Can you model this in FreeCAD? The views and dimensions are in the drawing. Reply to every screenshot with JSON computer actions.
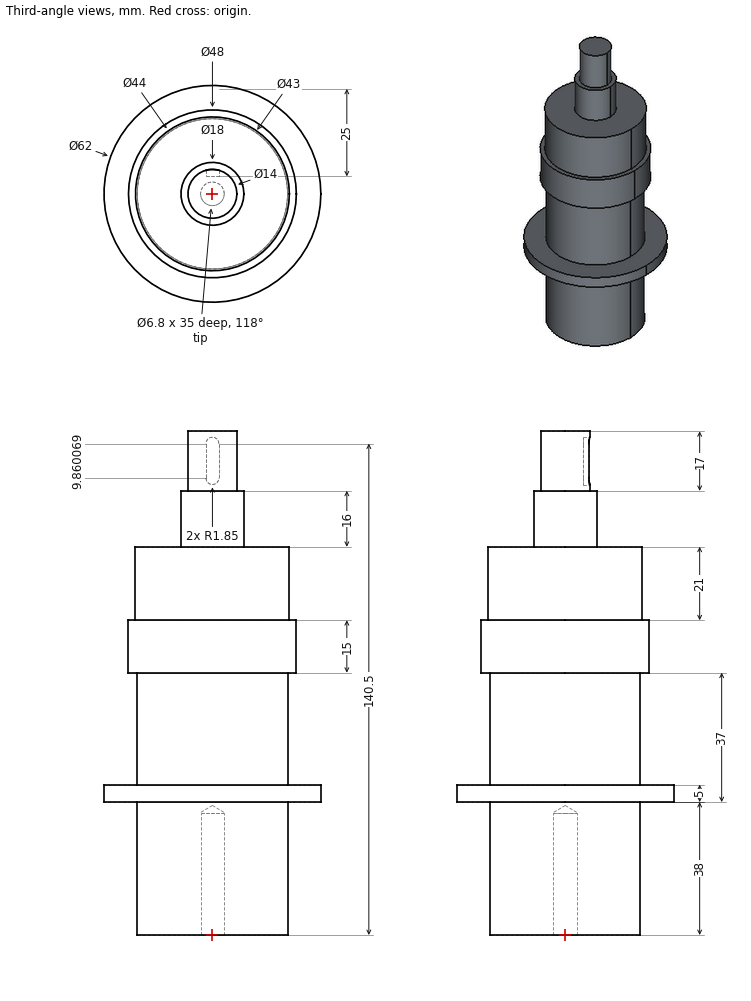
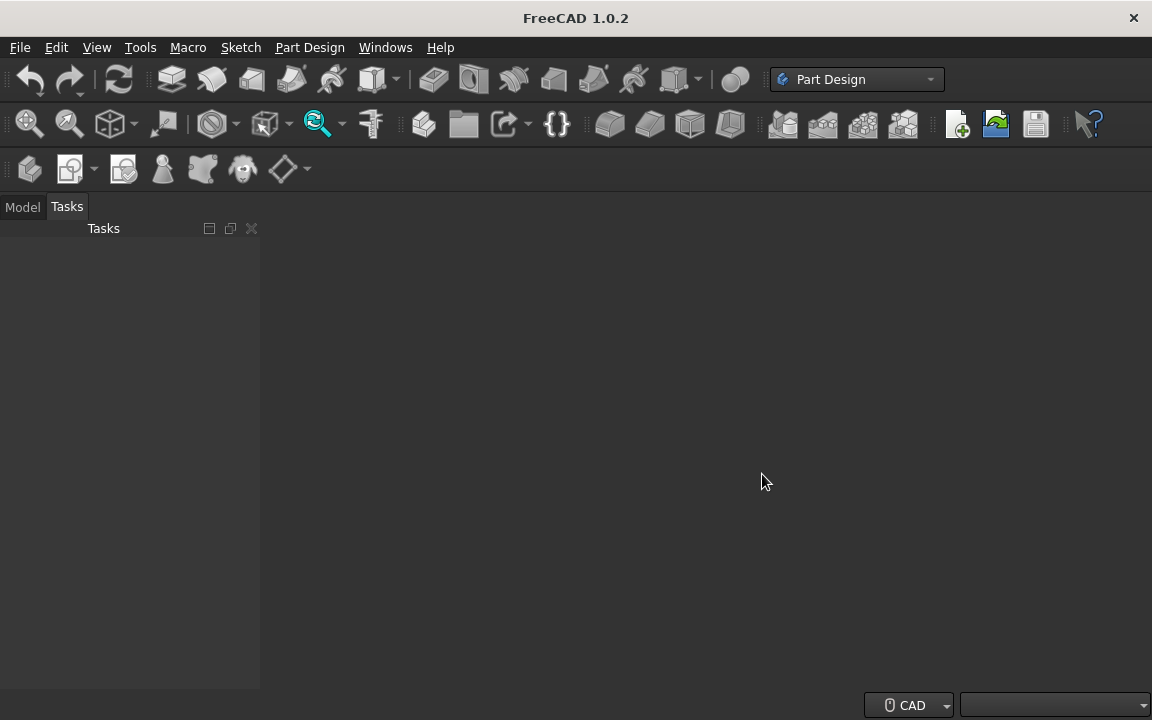
{"action": "left_click", "coordinate": [956, 124]}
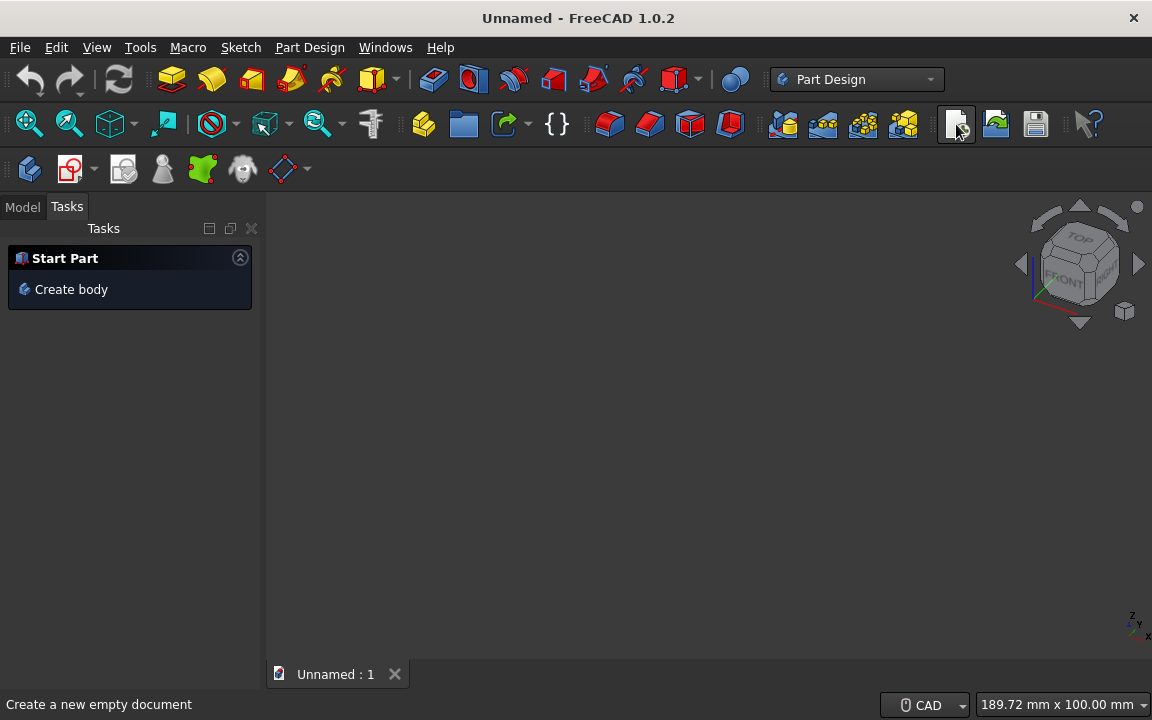
{"action": "left_click", "coordinate": [30, 170]}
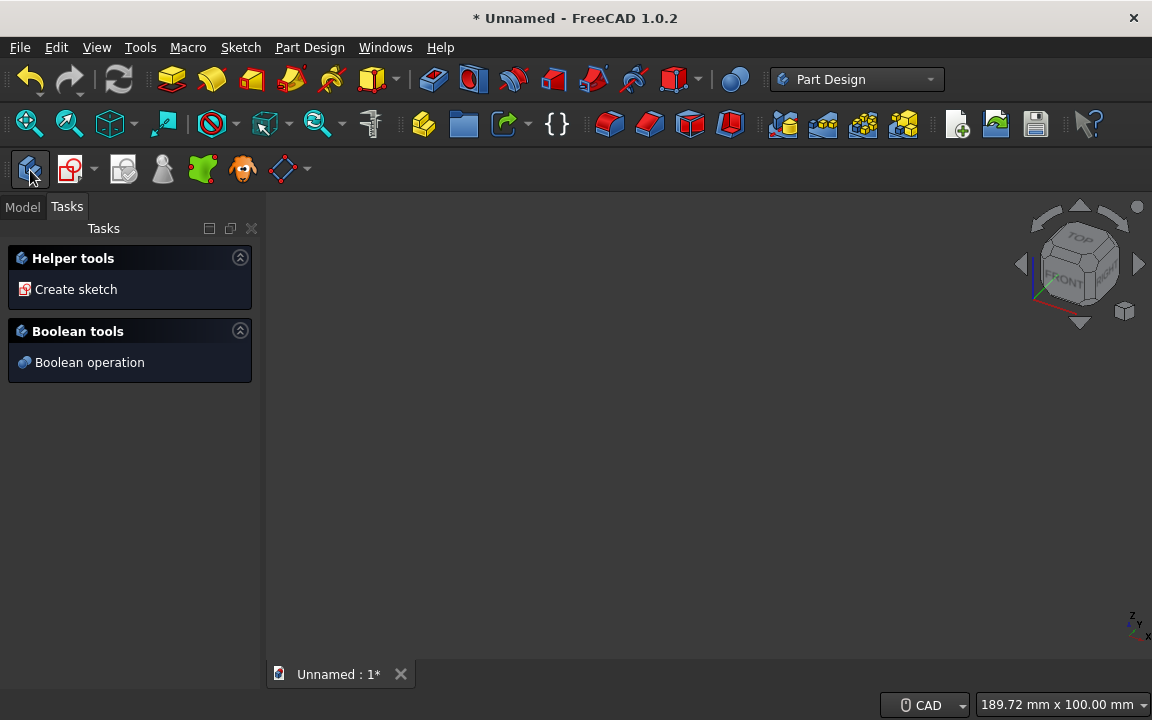
{"action": "left_click", "coordinate": [23, 206]}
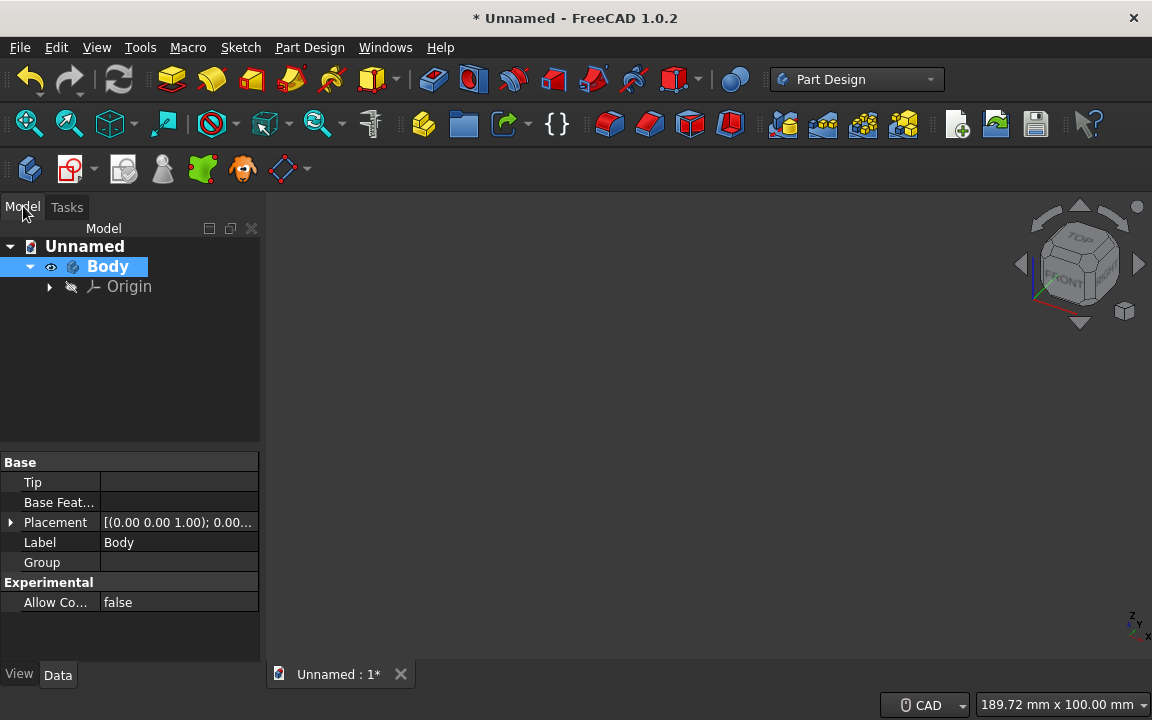
{"action": "left_click", "coordinate": [50, 287]}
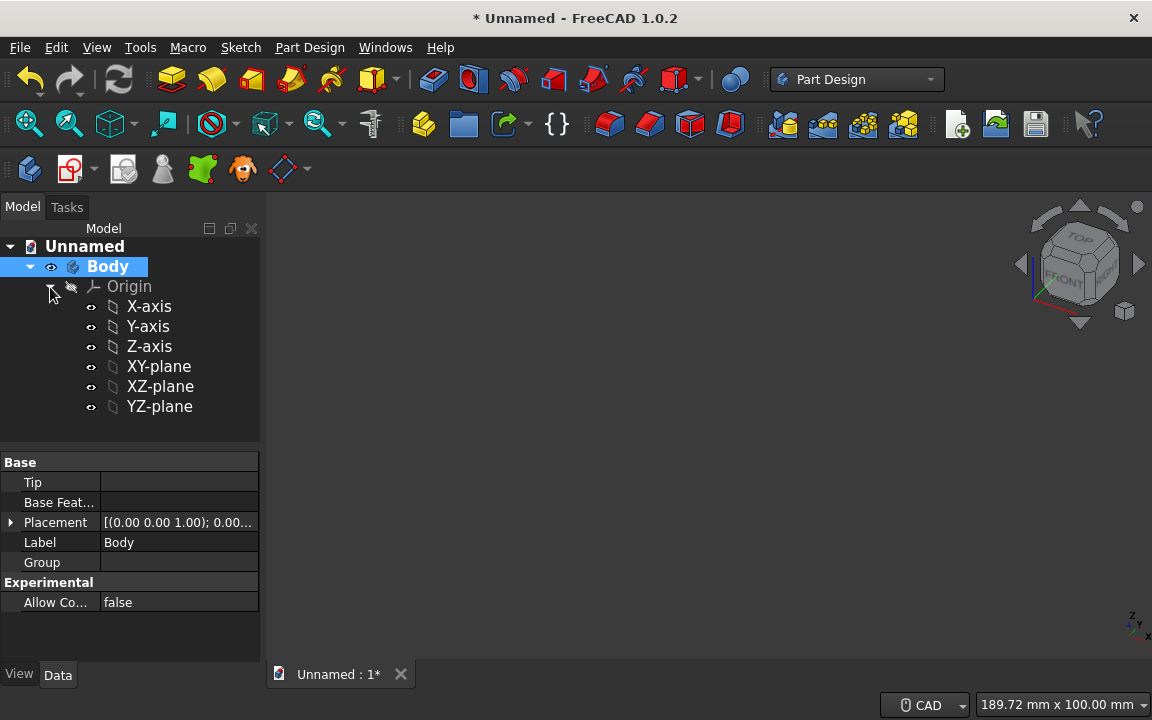
{"action": "left_click", "coordinate": [136, 367]}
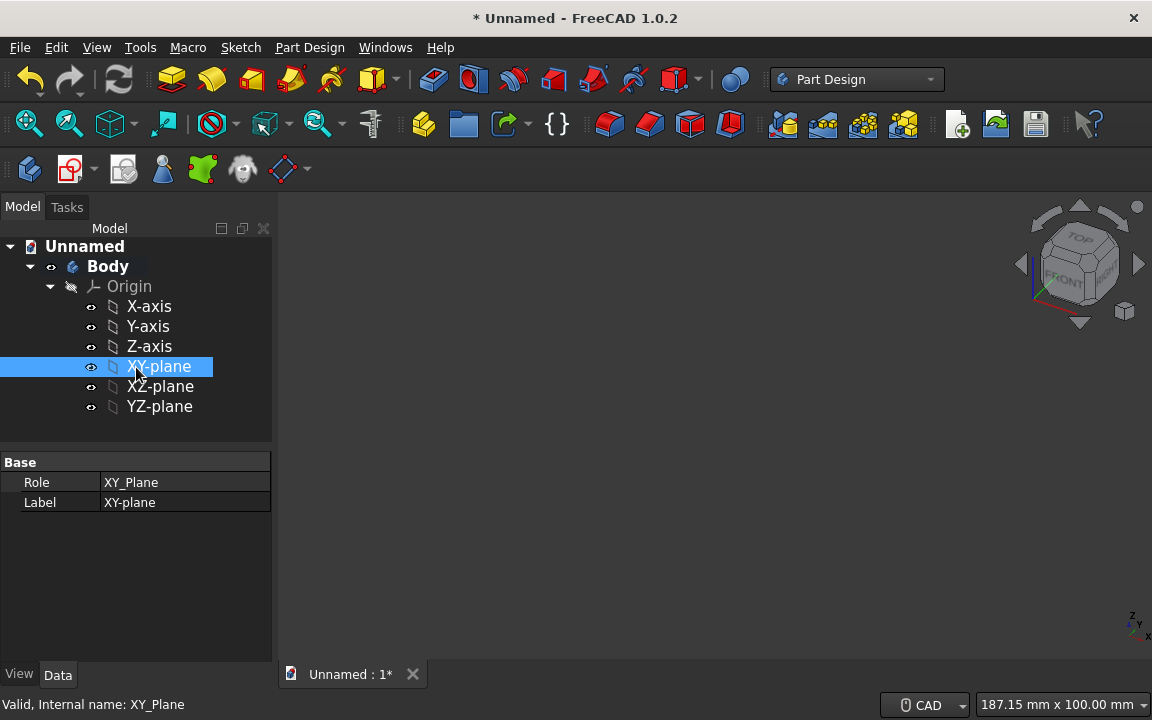
{"action": "left_click", "coordinate": [284, 170]}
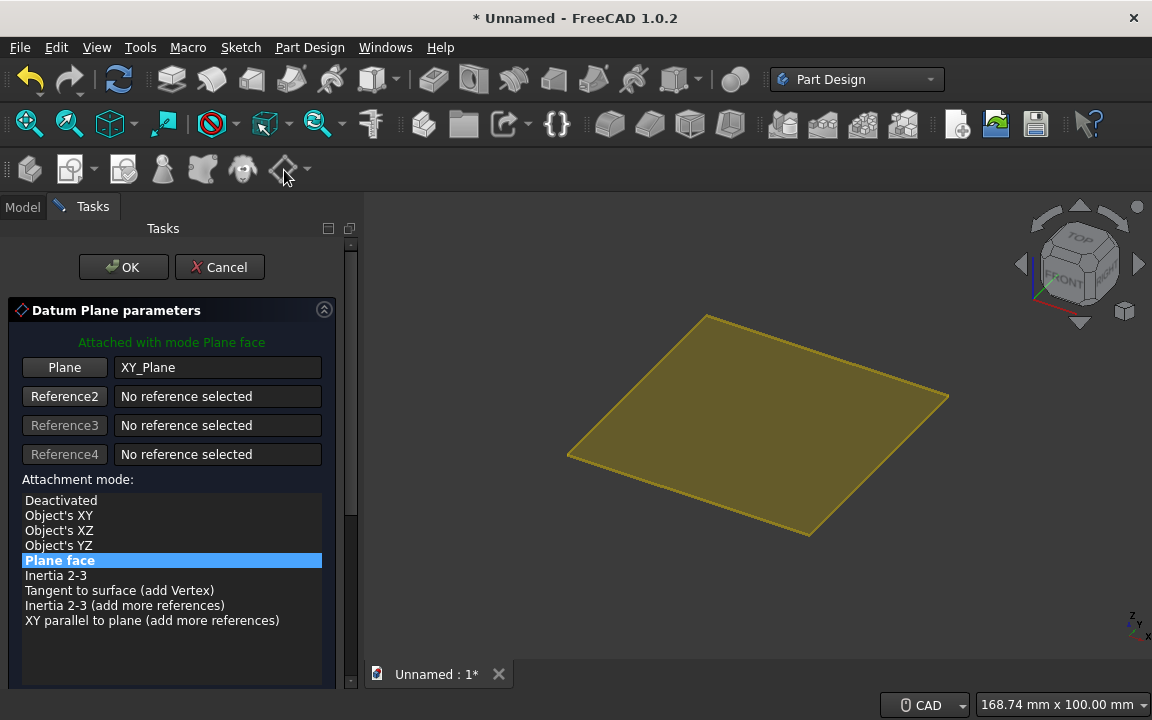
{"action": "scroll", "coordinate": [351, 463], "scroll_direction": "down", "scroll_amount": 3}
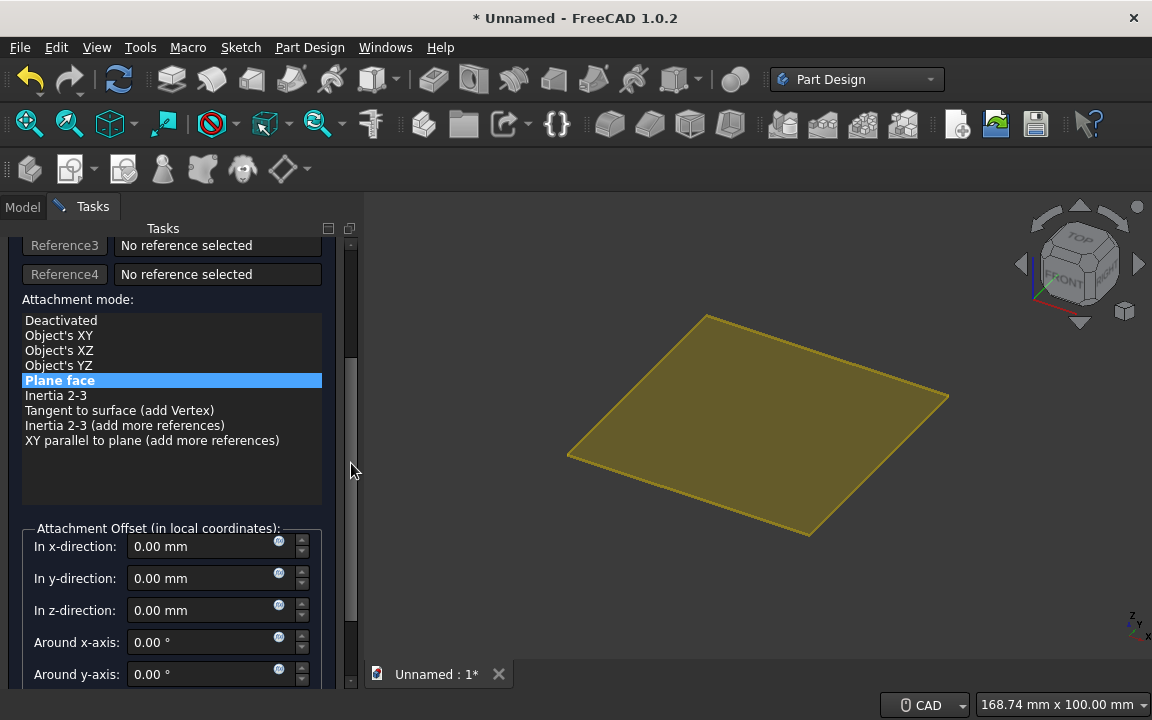
{"action": "triple_click", "coordinate": [210, 610]}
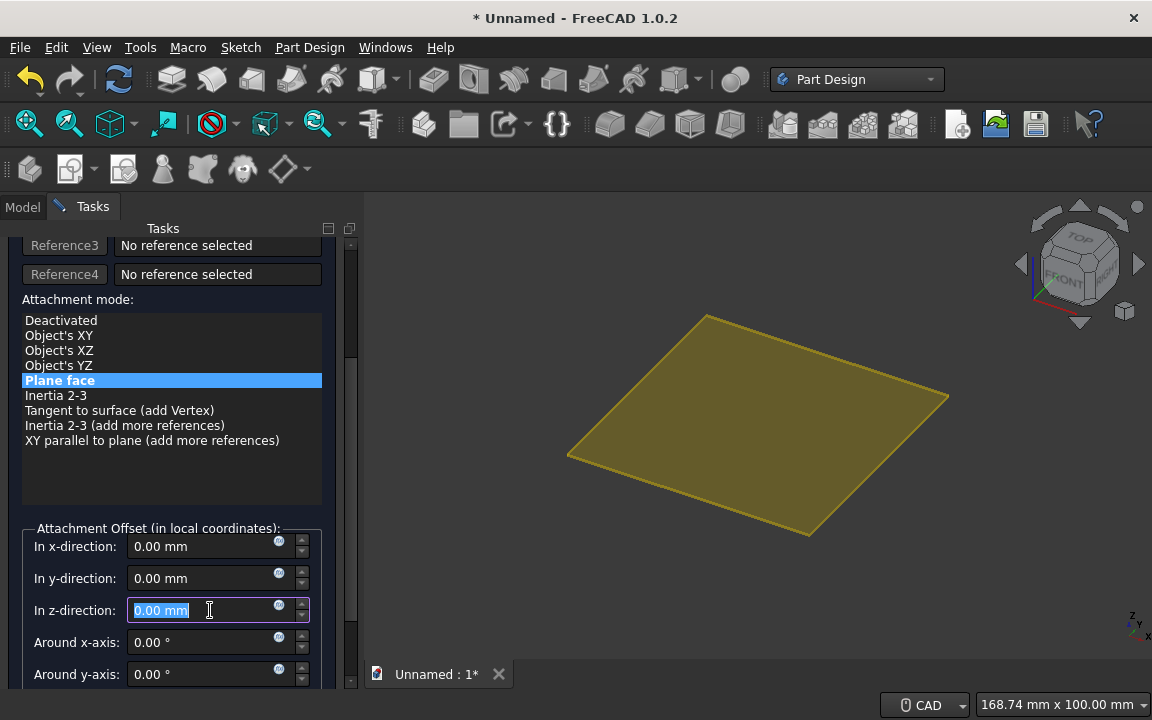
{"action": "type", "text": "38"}
{"action": "key", "text": "Tab"}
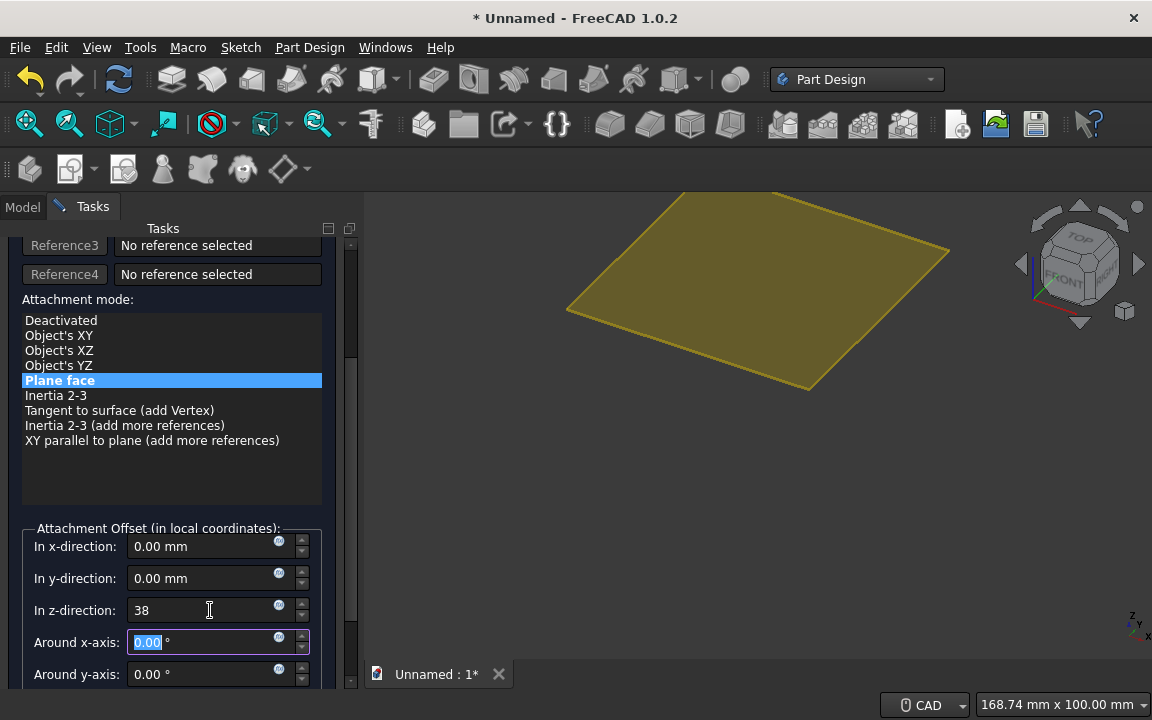
{"action": "scroll", "coordinate": [351, 463], "scroll_direction": "up", "scroll_amount": 4}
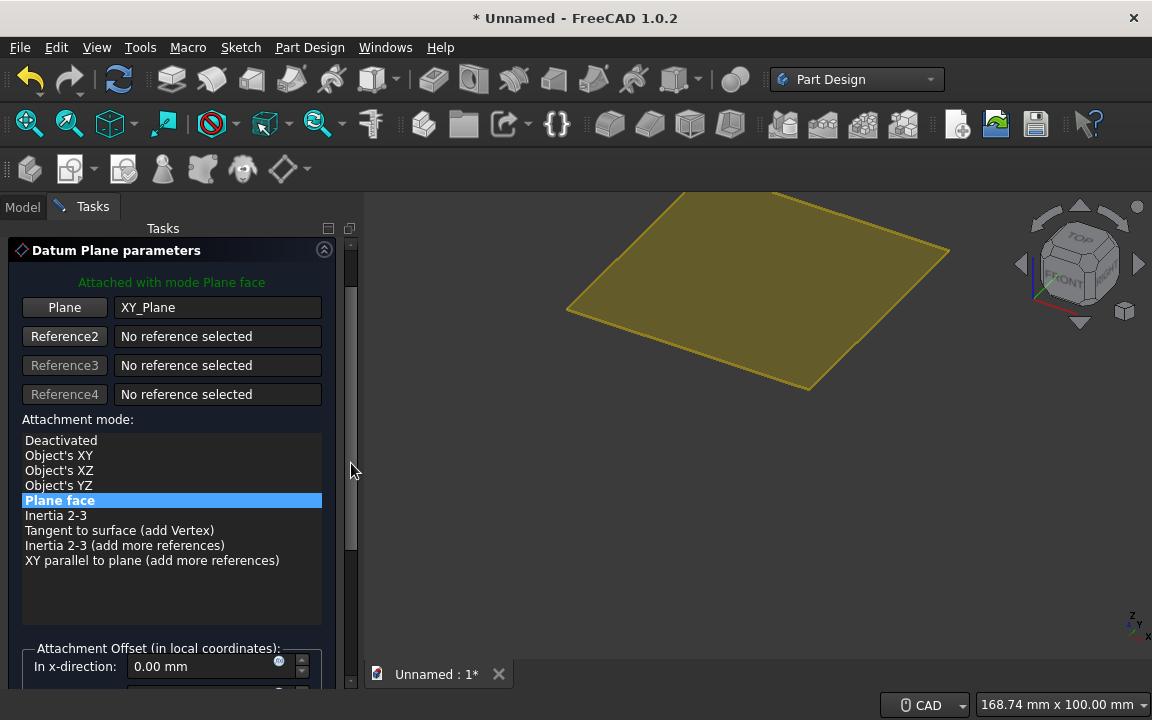
{"action": "left_click", "coordinate": [124, 267]}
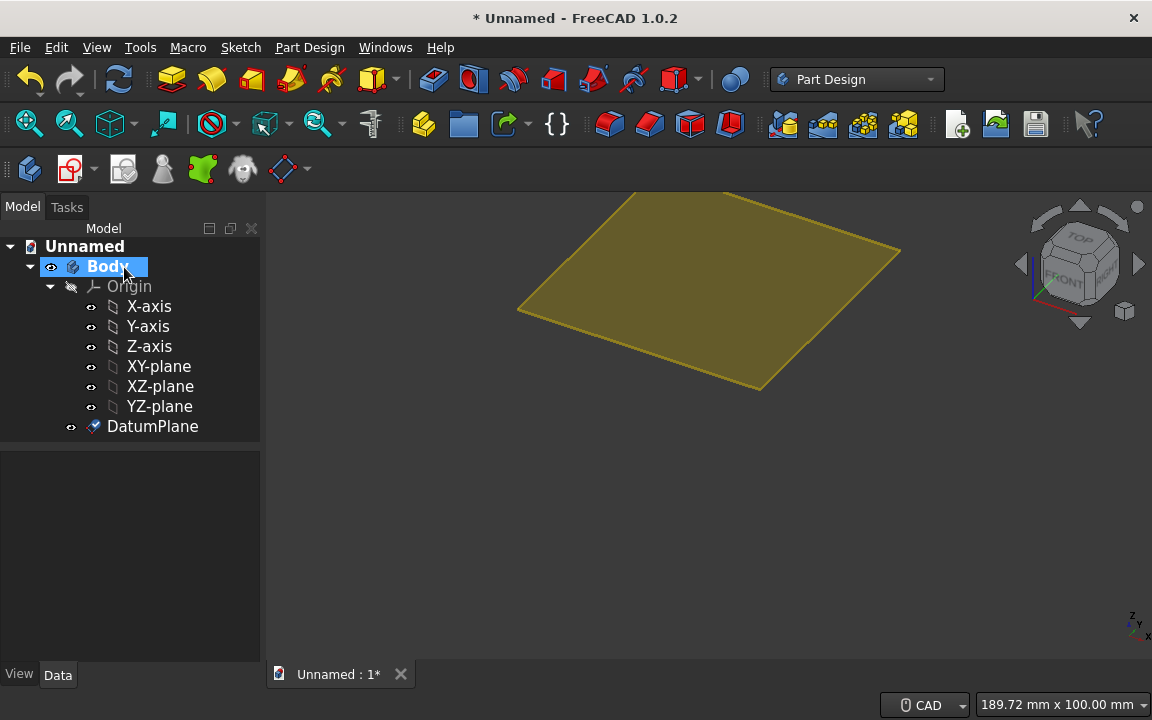
{"action": "left_click", "coordinate": [116, 427]}